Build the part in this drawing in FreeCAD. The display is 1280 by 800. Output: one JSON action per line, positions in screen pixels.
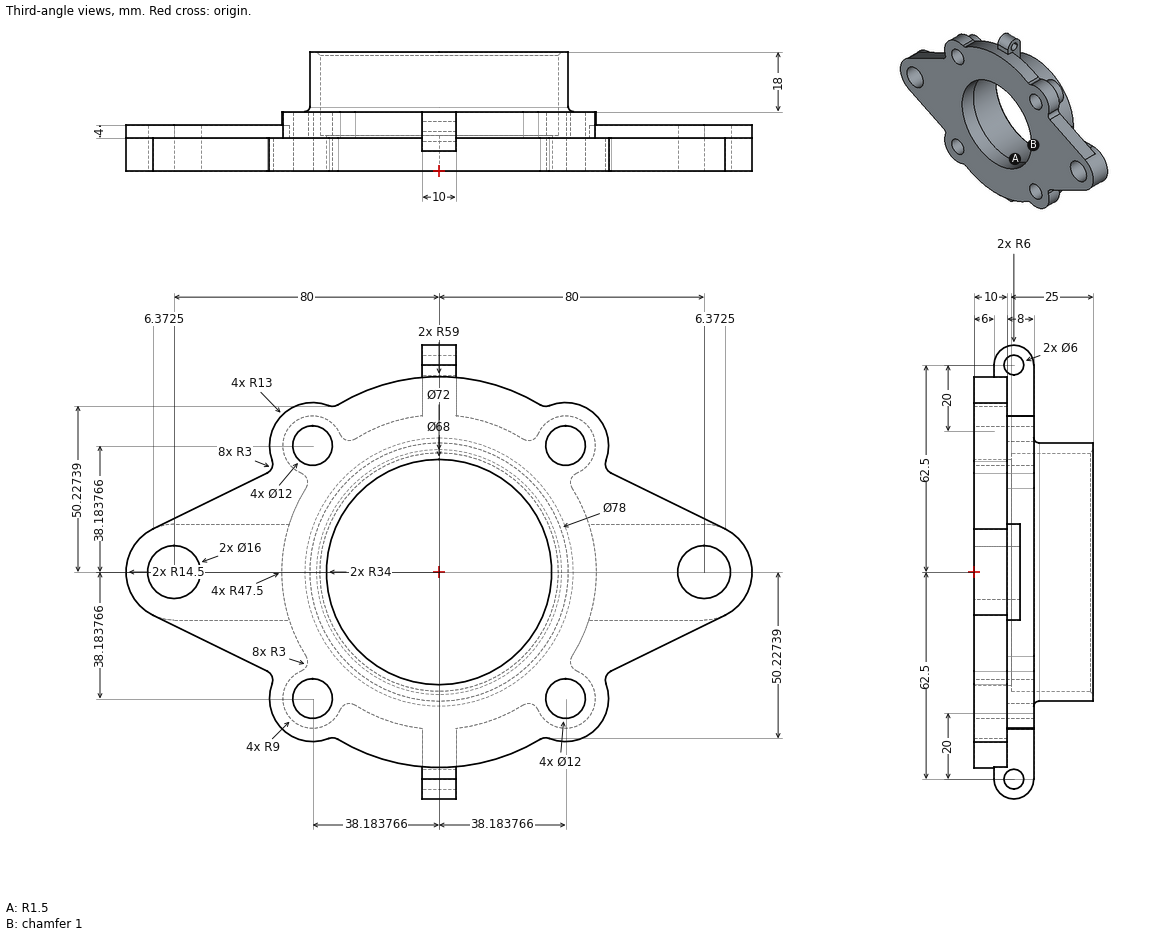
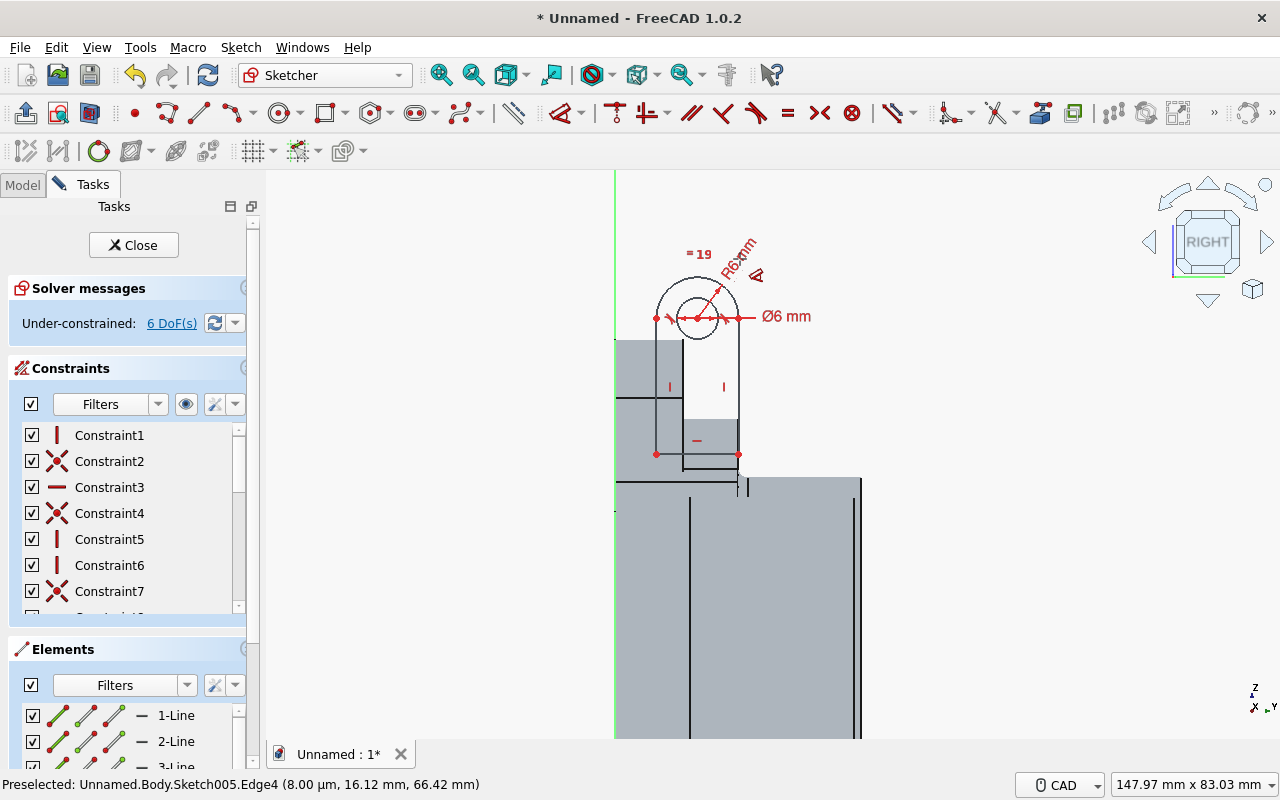
{"action": "left_click", "coordinate": [656, 359]}
{"action": "left_click", "coordinate": [690, 386]}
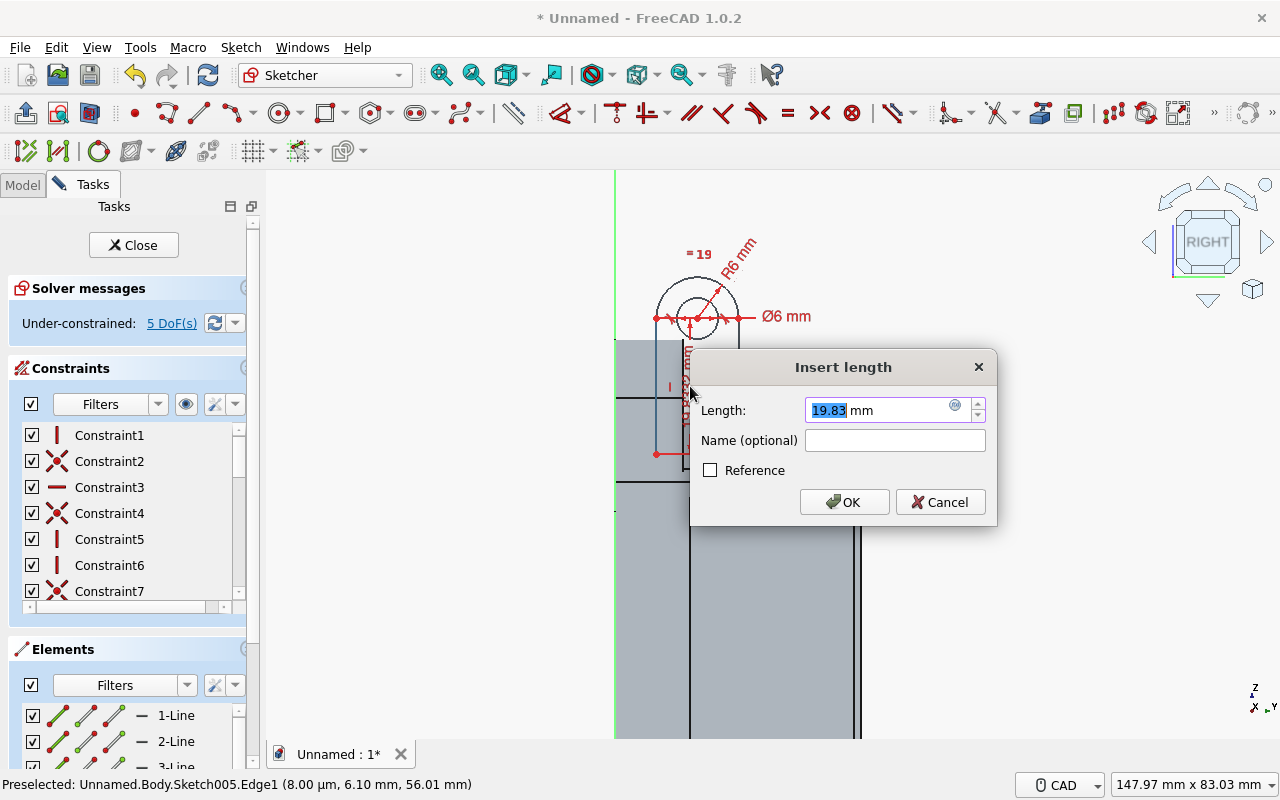
{"action": "type", "text": "20"}
{"action": "key", "text": "Return"}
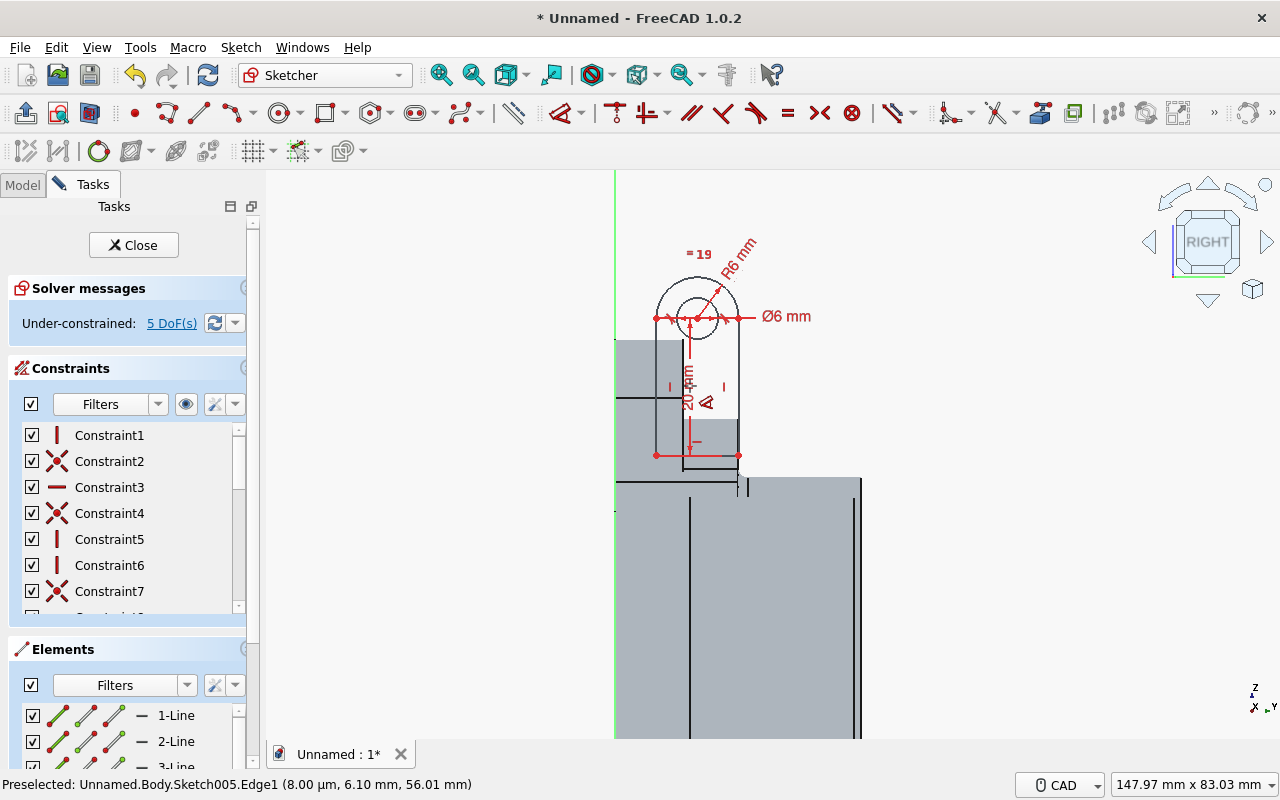
{"action": "scroll", "coordinate": [721, 286], "scroll_direction": "down", "scroll_amount": 5}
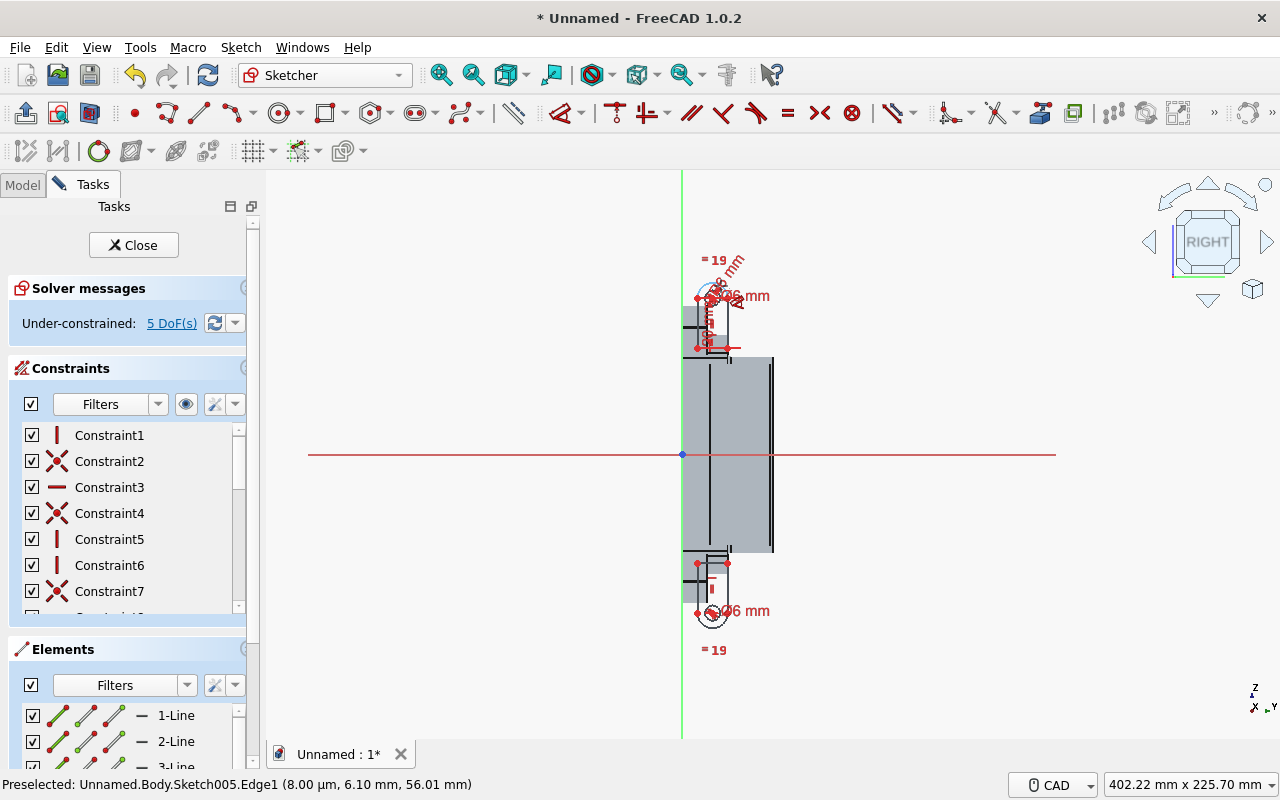
{"action": "left_click", "coordinate": [728, 598]}
{"action": "left_click", "coordinate": [762, 588]}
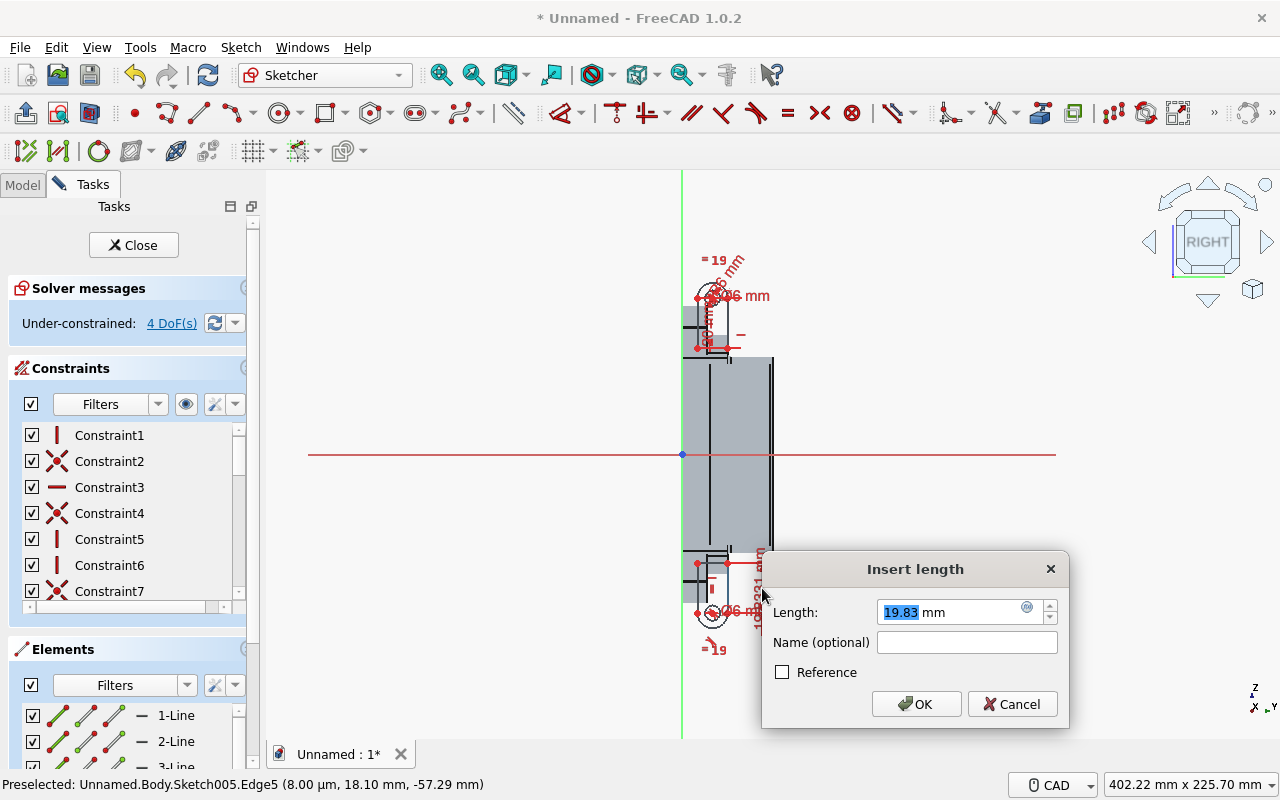
{"action": "type", "text": "20"}
{"action": "key", "text": "Return"}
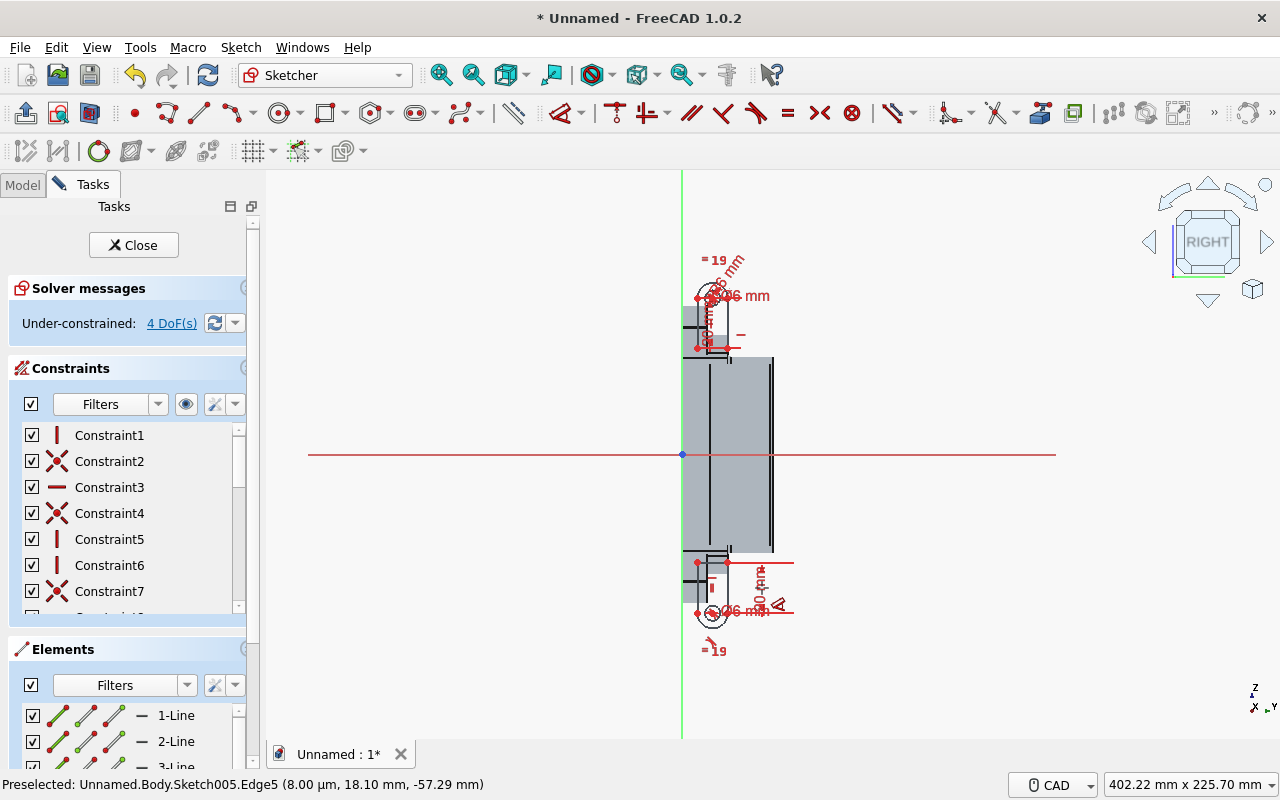
{"action": "scroll", "coordinate": [698, 298], "scroll_direction": "up", "scroll_amount": 5}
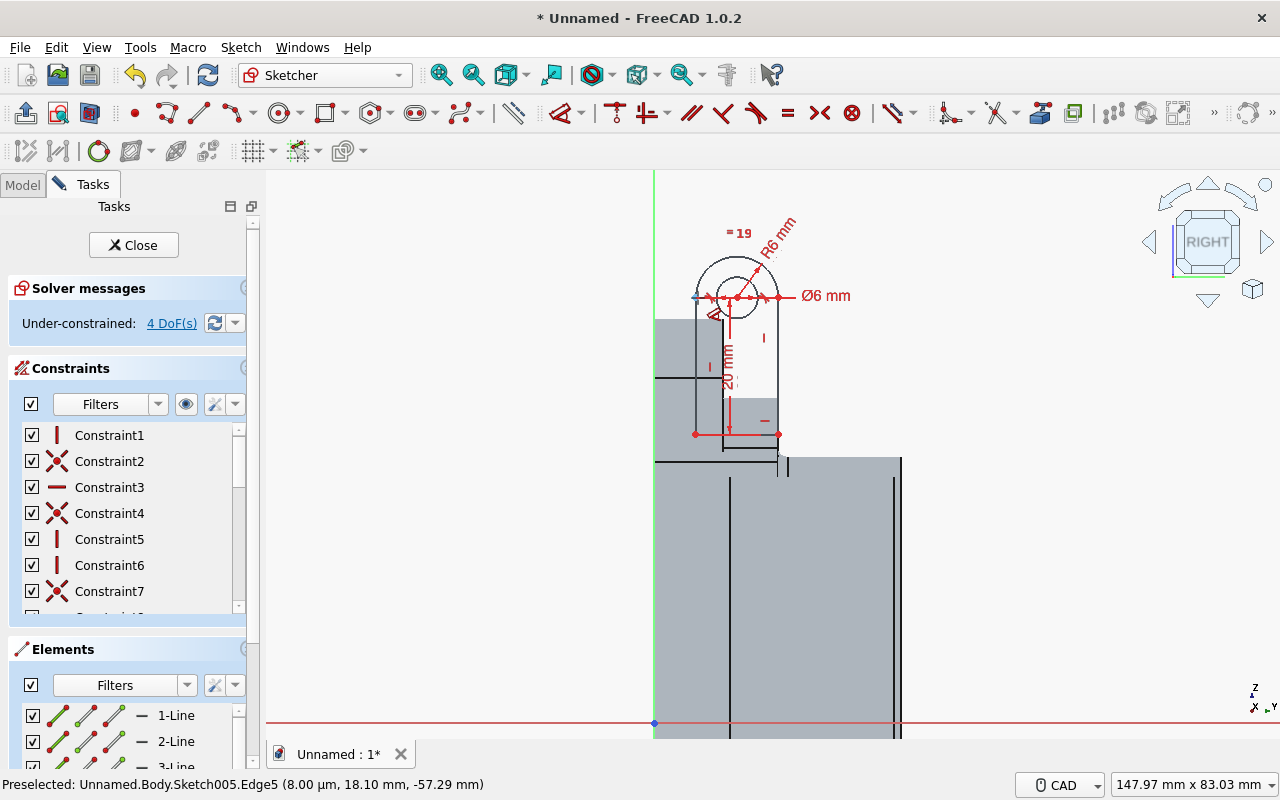
{"action": "left_click", "coordinate": [696, 298]}
{"action": "left_click", "coordinate": [675, 264]}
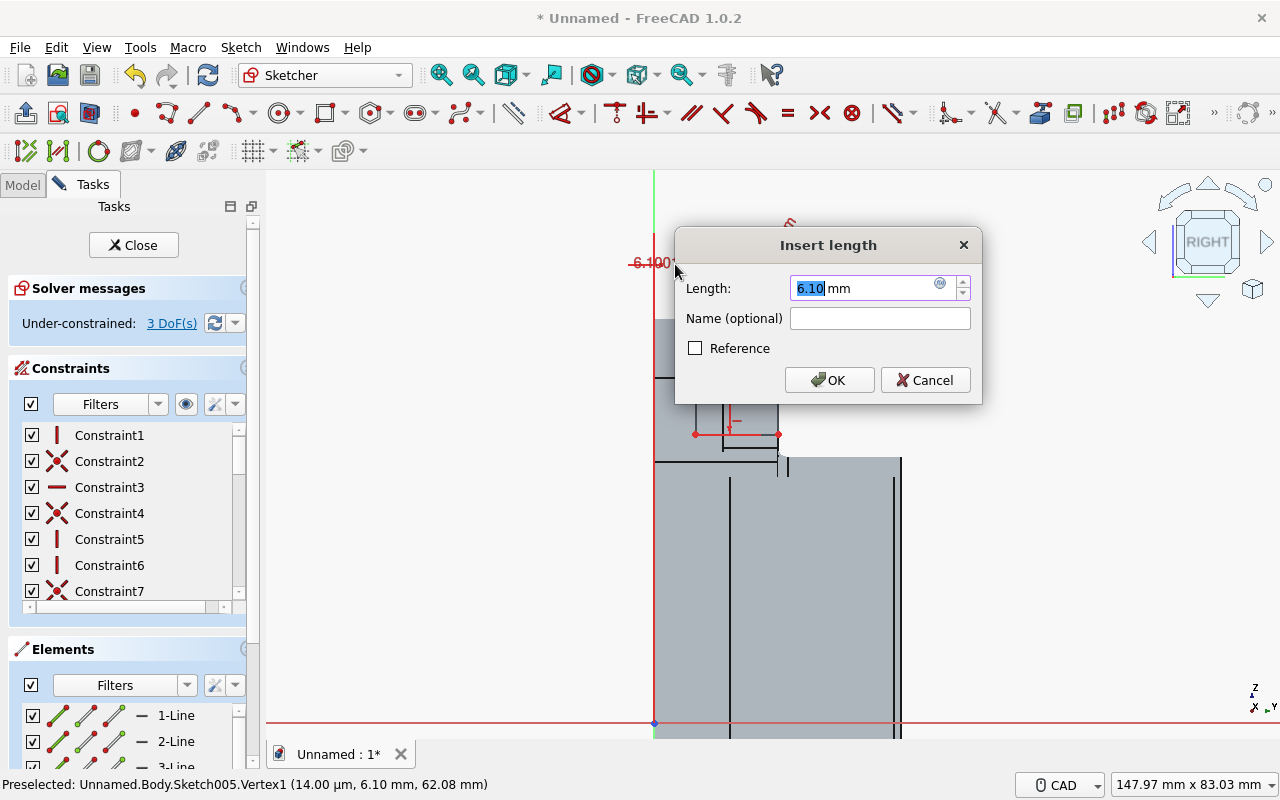
{"action": "type", "text": "6"}
{"action": "key", "text": "Return"}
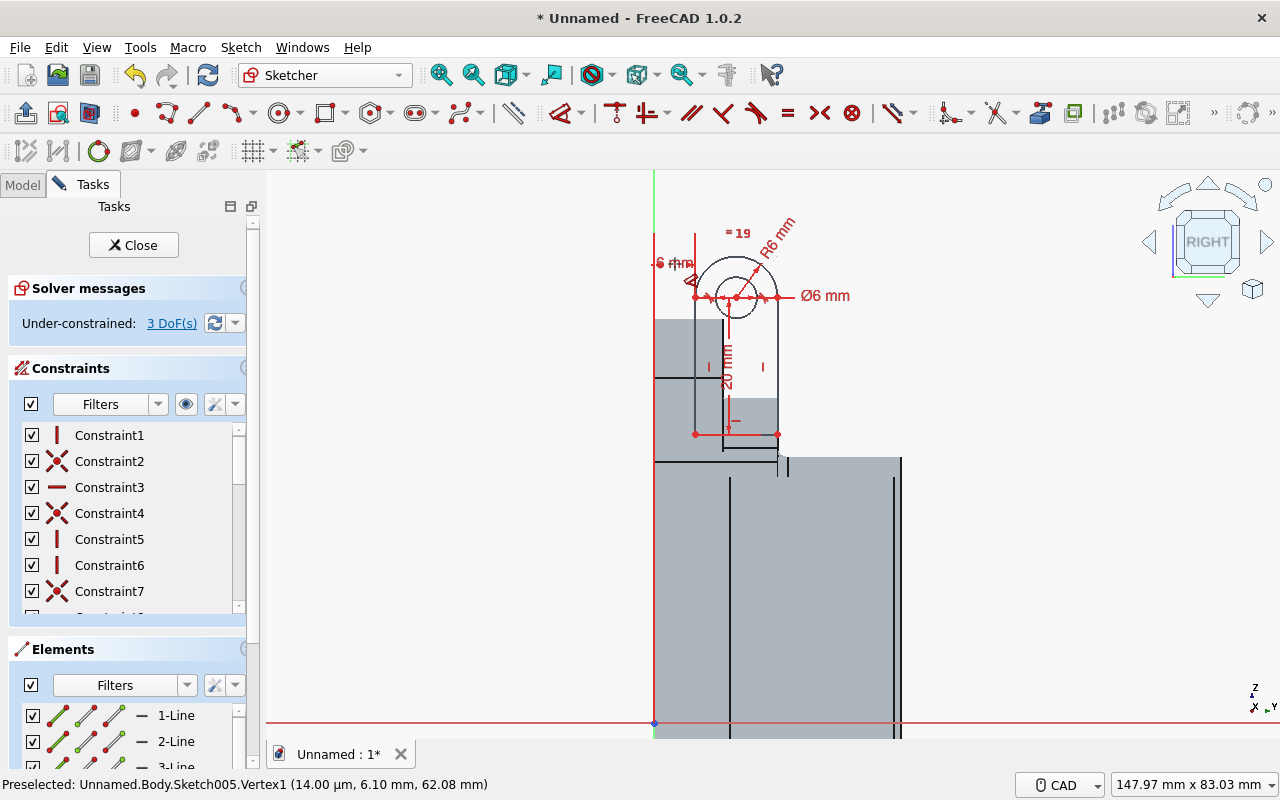
{"action": "scroll", "coordinate": [698, 298], "scroll_direction": "down", "scroll_amount": 5}